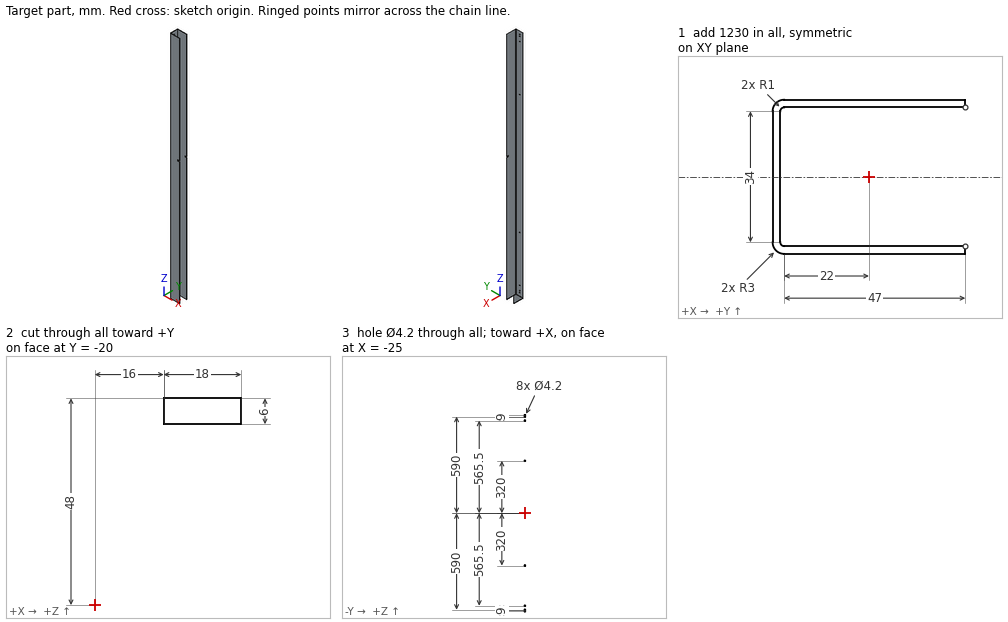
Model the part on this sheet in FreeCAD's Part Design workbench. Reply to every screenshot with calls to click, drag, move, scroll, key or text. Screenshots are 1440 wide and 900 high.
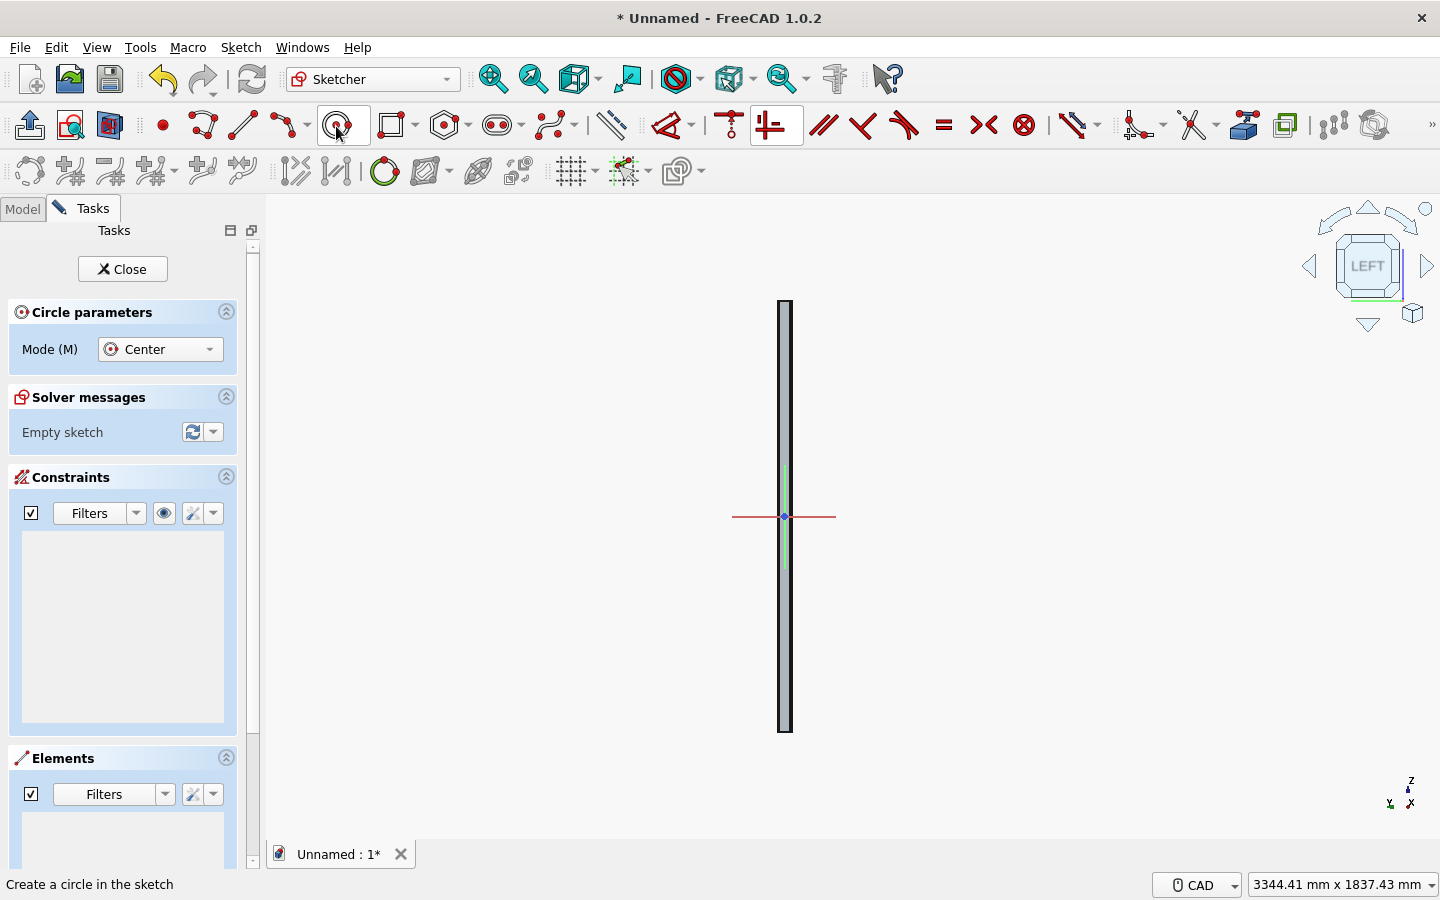
scroll(785, 309, up, 18)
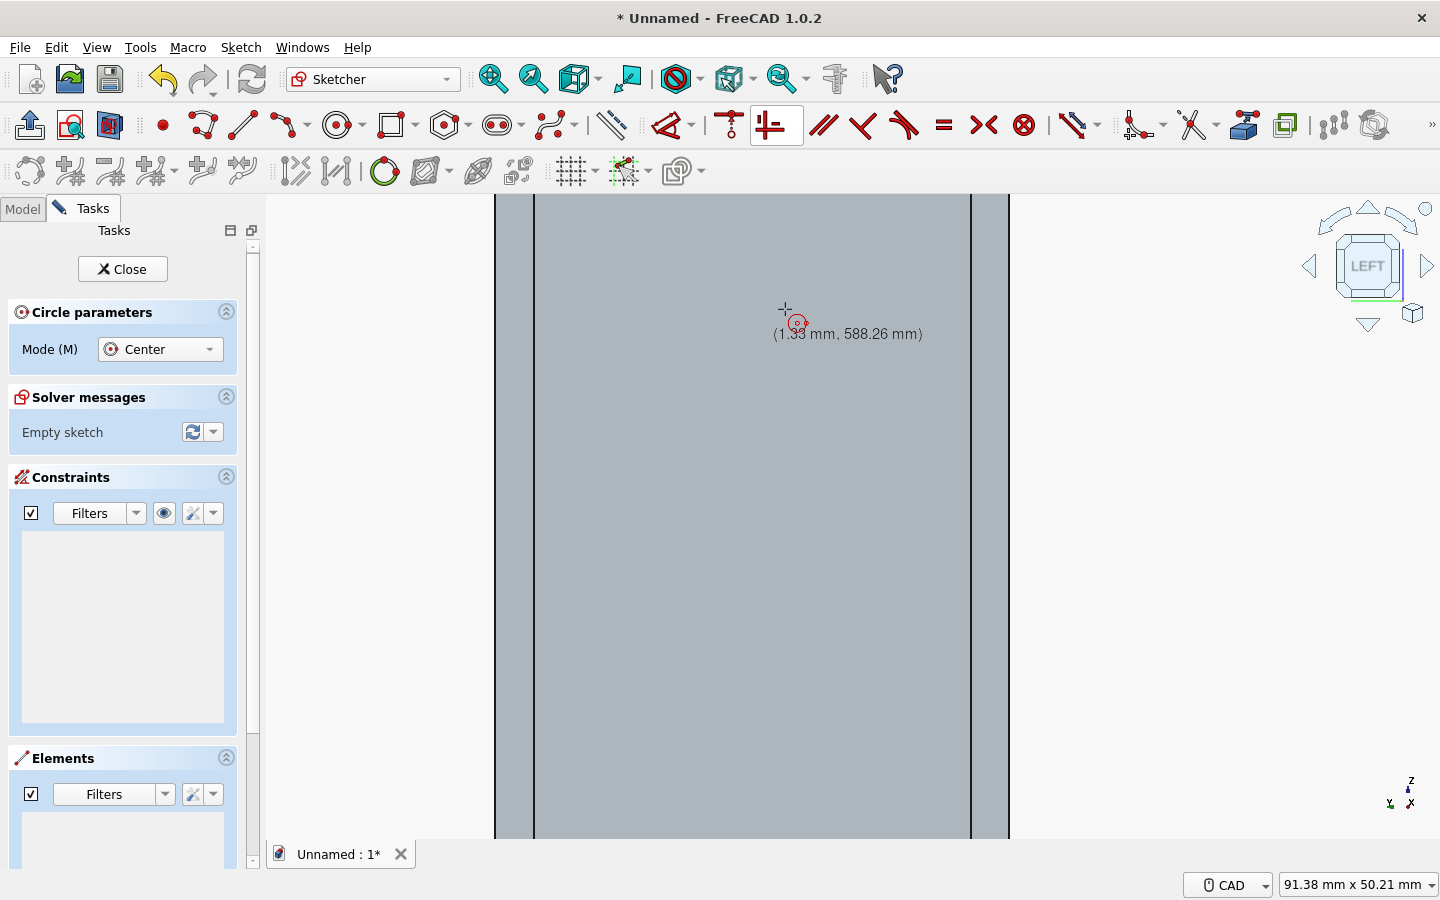
scroll(786, 262, down, 17)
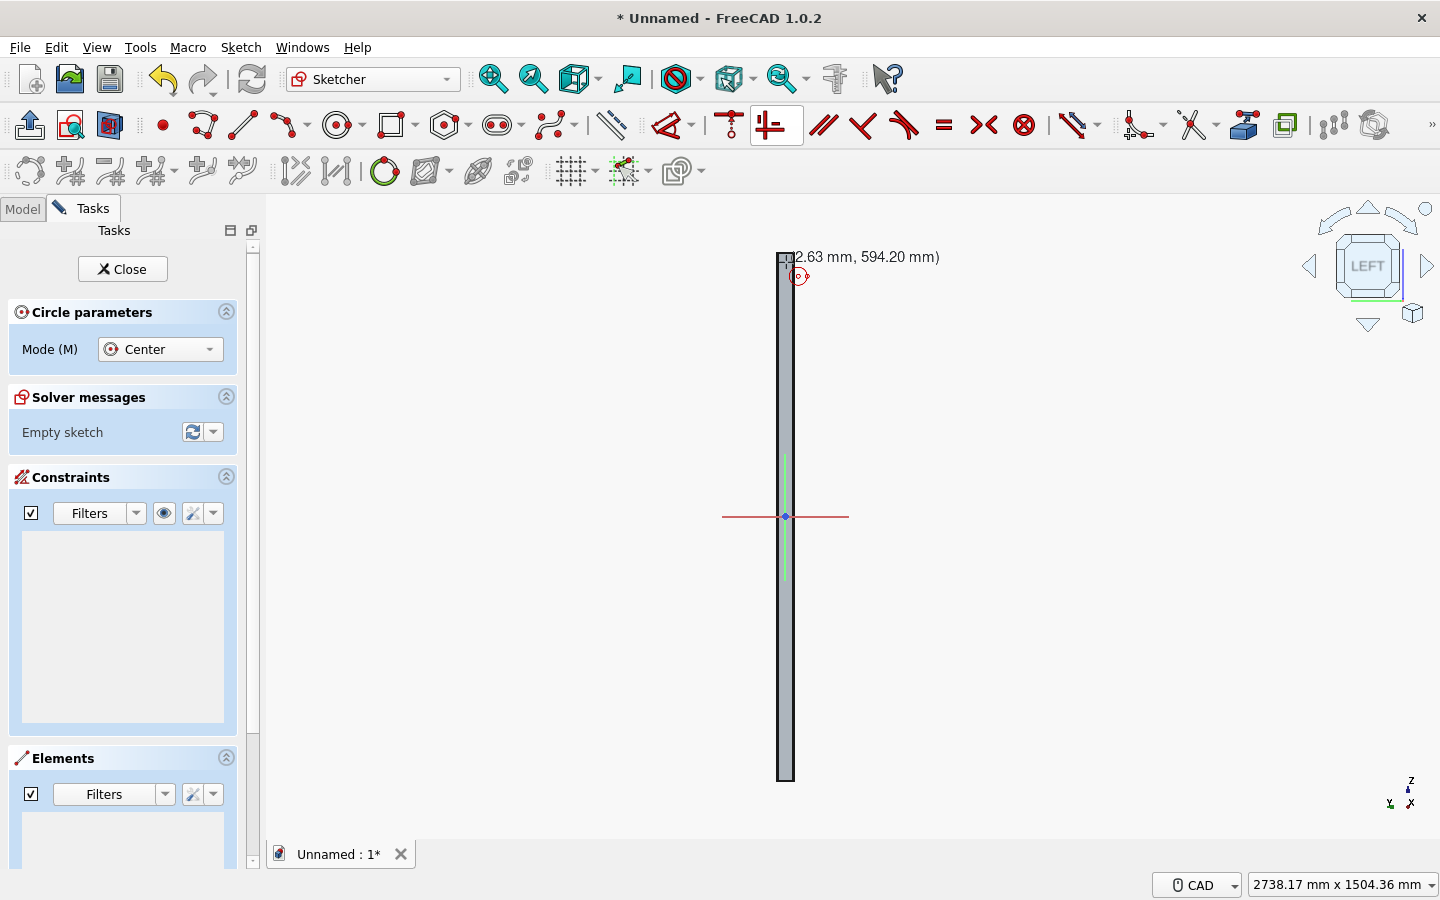
click(785, 264)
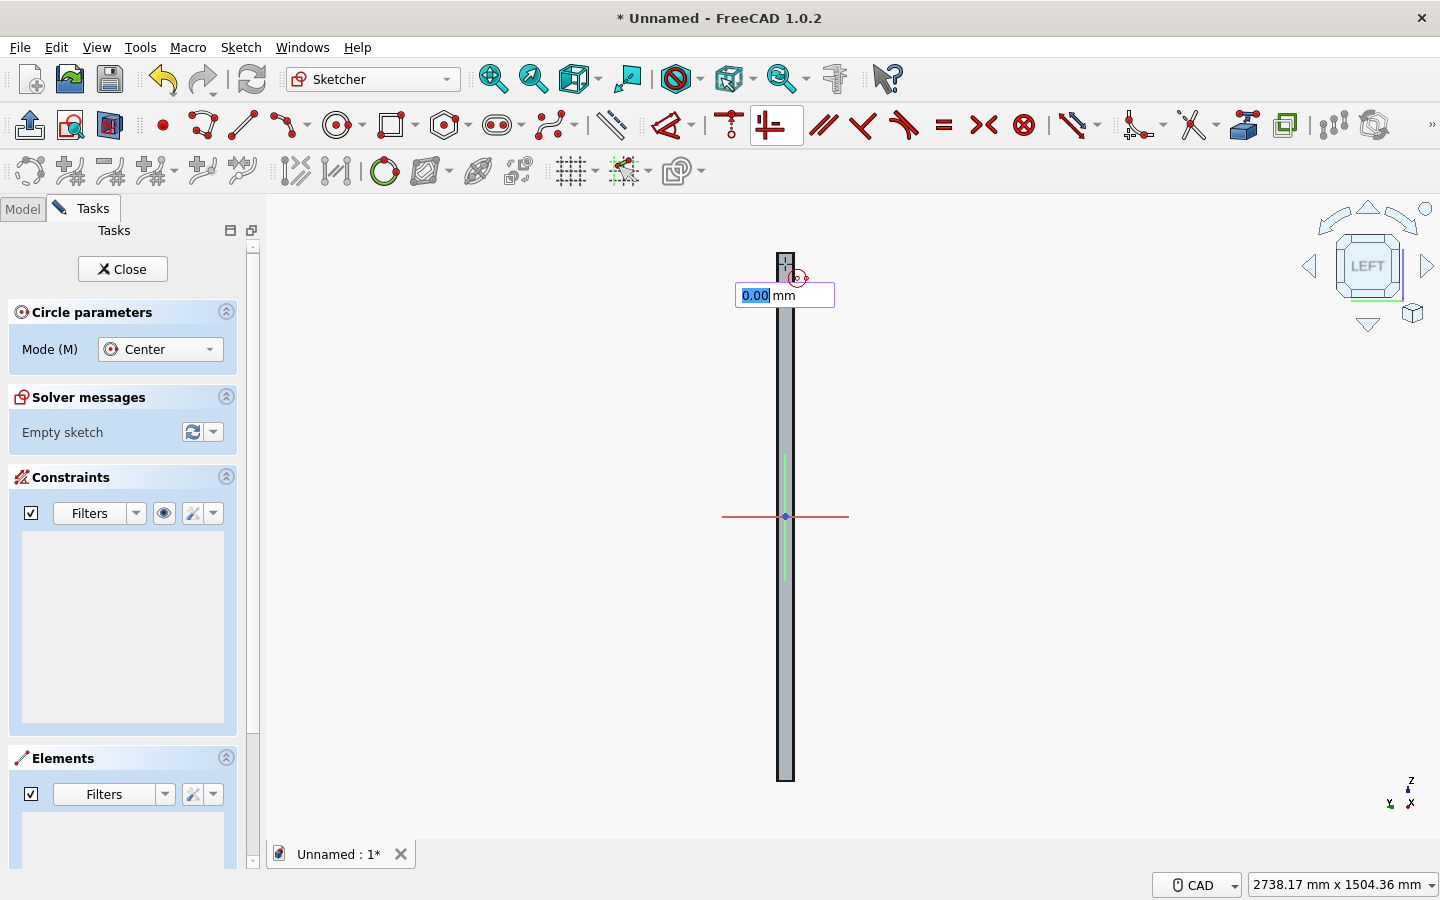
scroll(786, 264, up, 15)
move(780, 254)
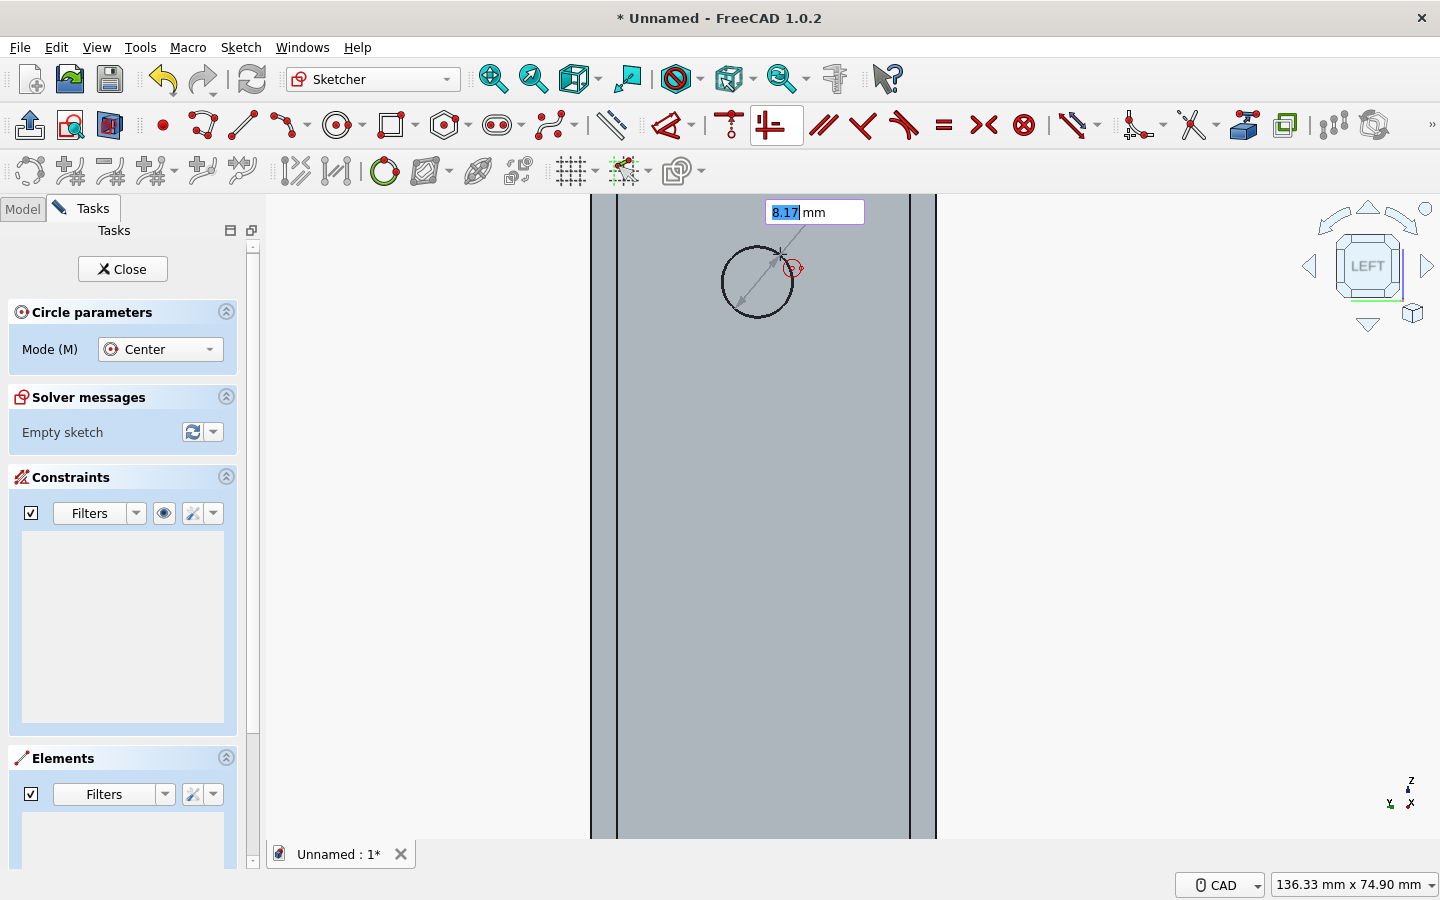
text(4.2)
key(Return)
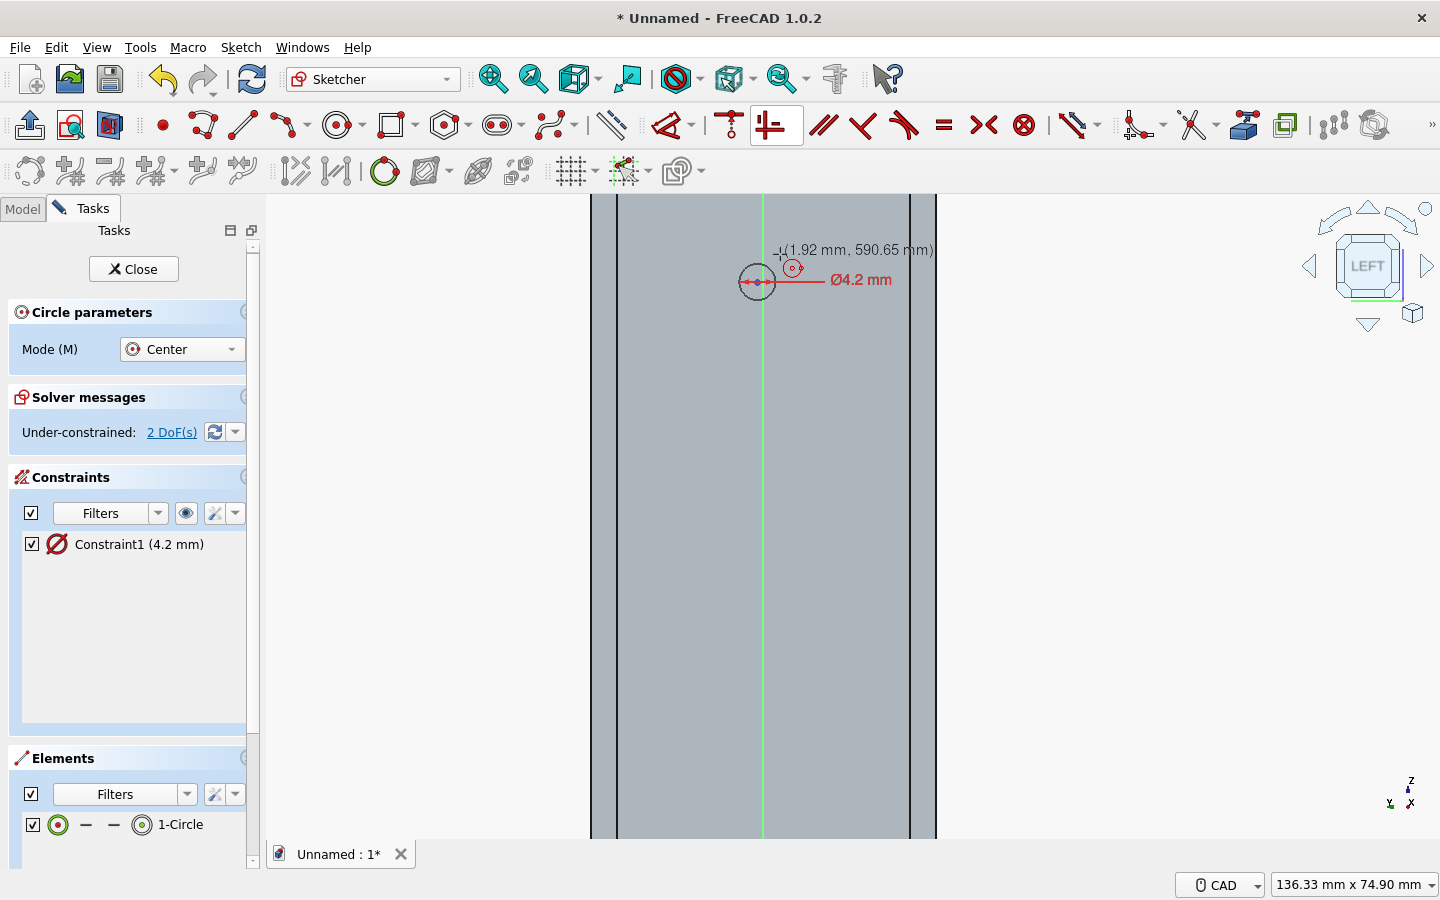
scroll(786, 264, down, 15)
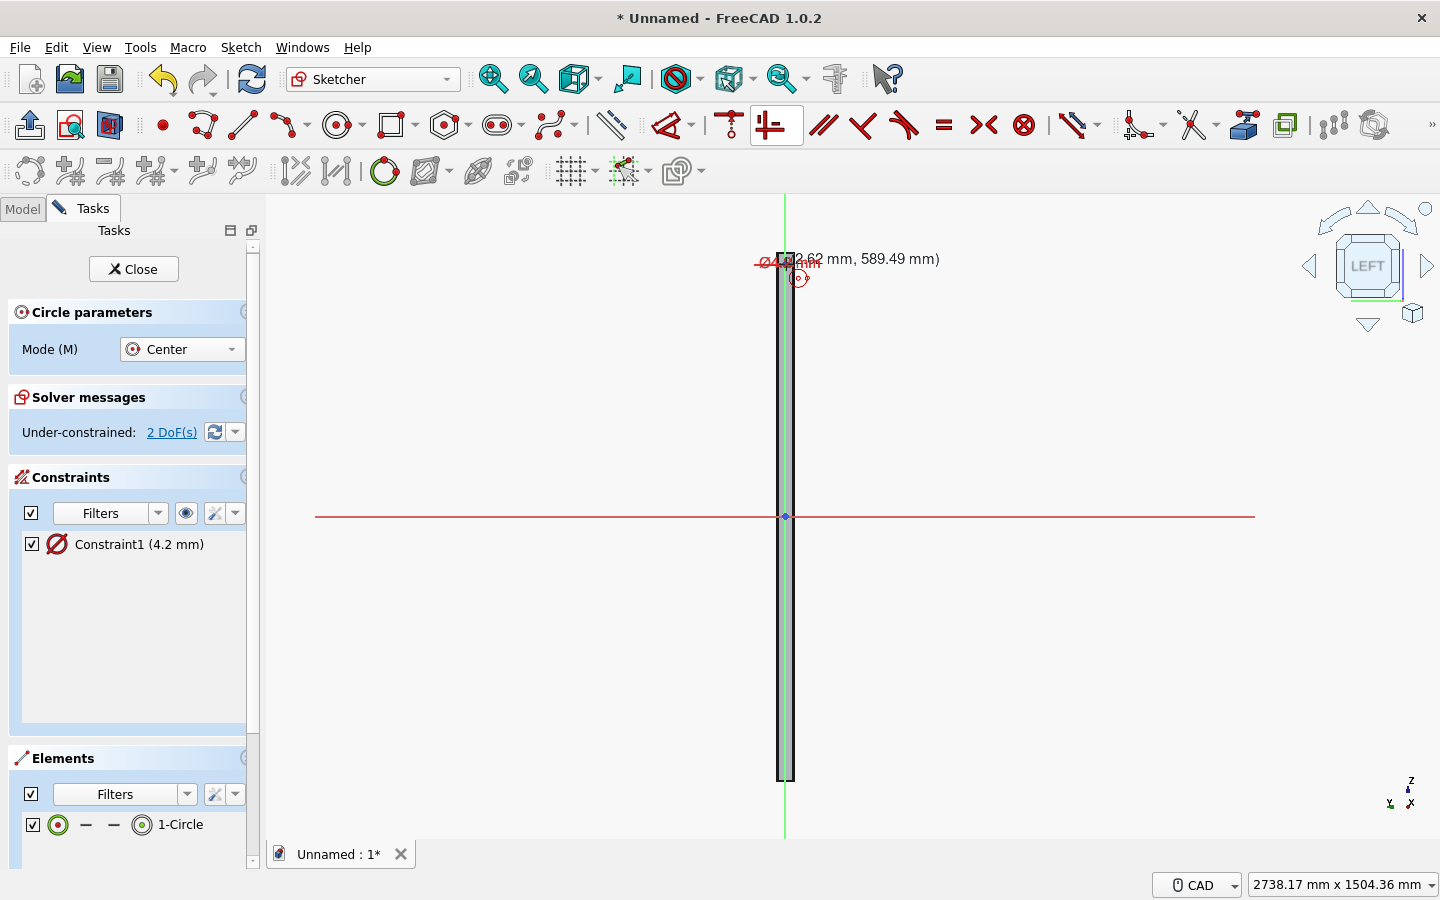
scroll(785, 380, up, 17)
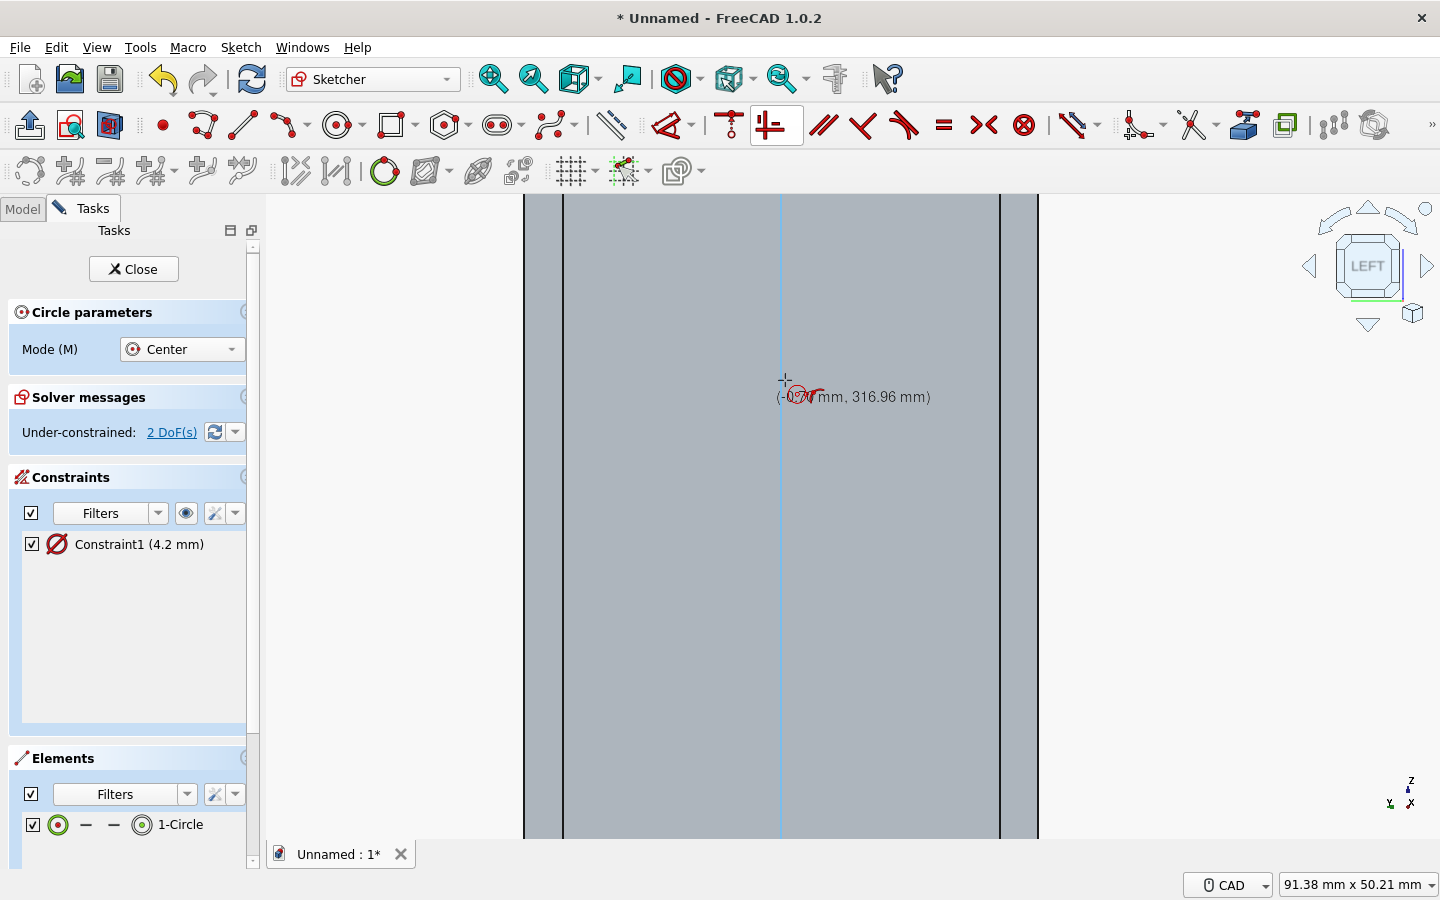
scroll(785, 380, down, 17)